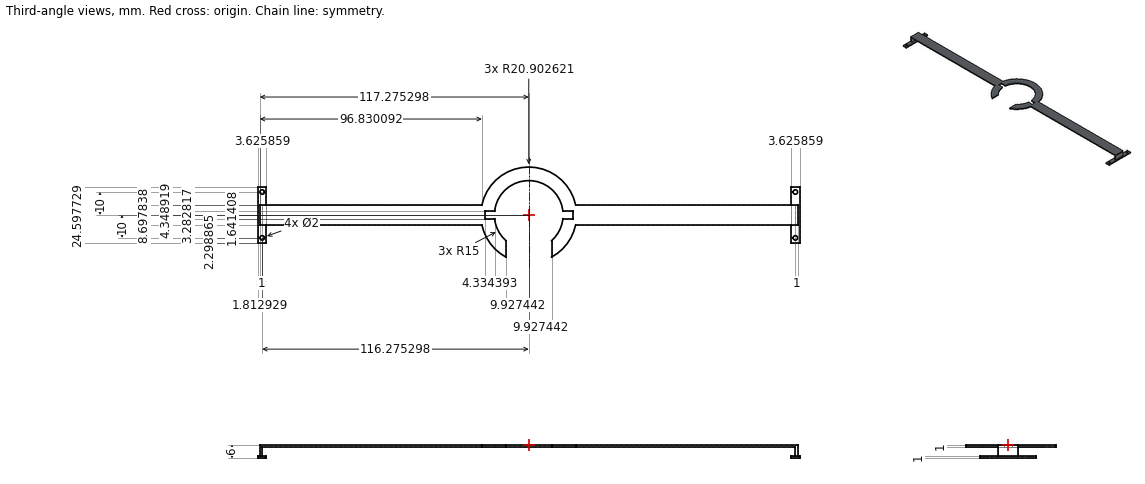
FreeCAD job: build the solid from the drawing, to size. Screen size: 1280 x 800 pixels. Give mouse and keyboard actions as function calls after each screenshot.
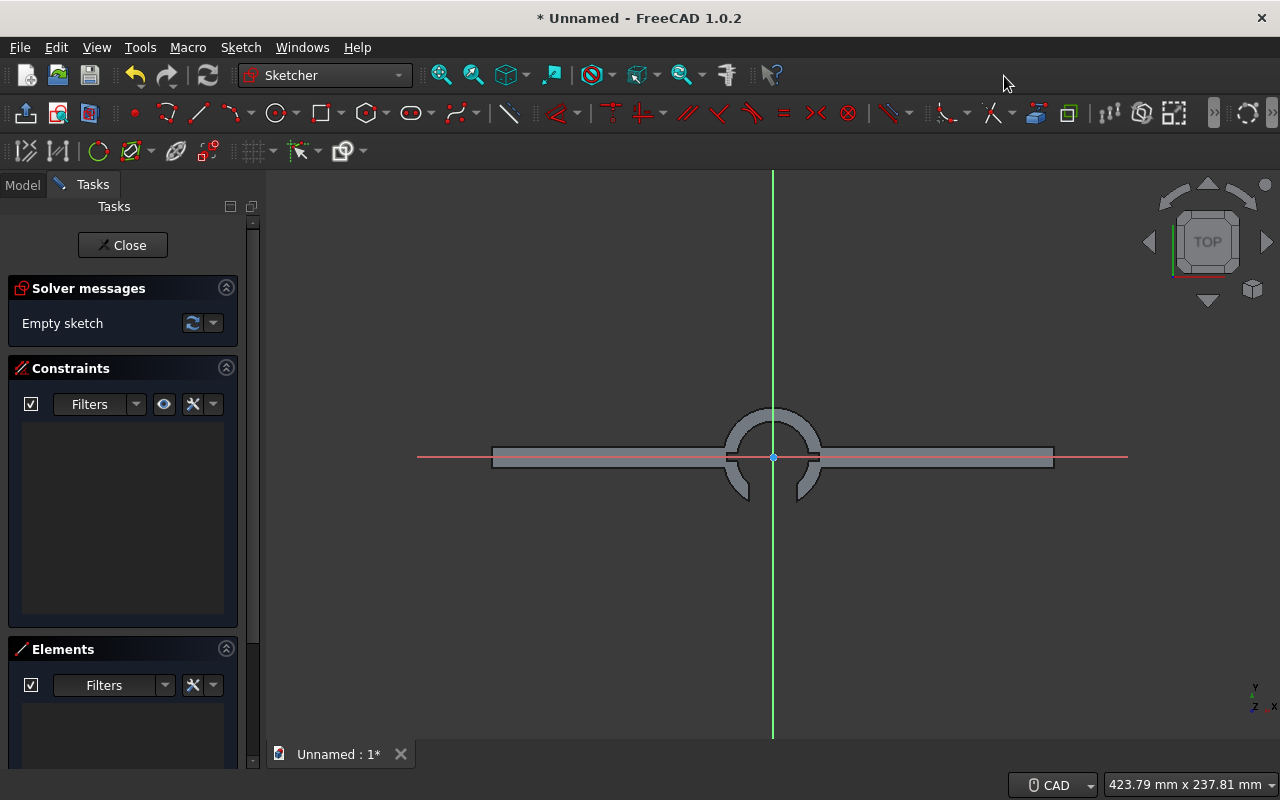
click(322, 114)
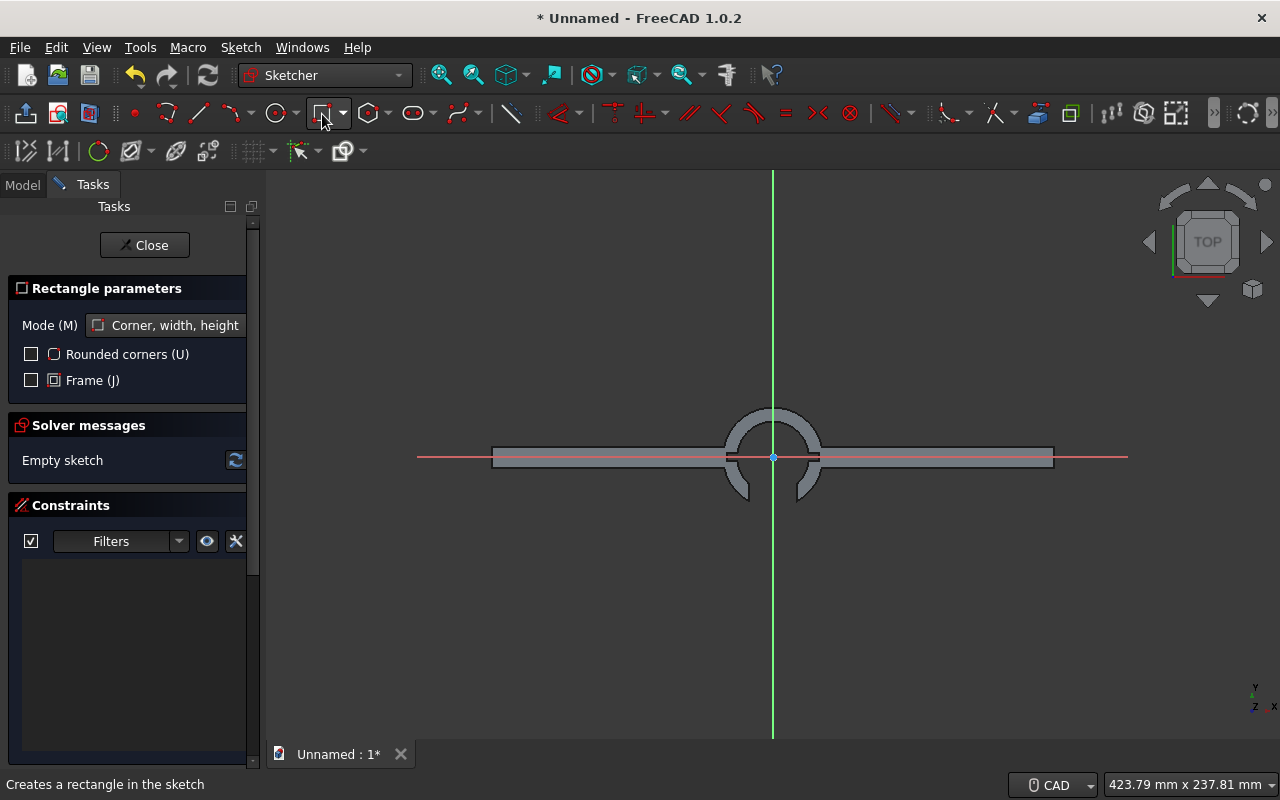
scroll(492, 447, up, 10)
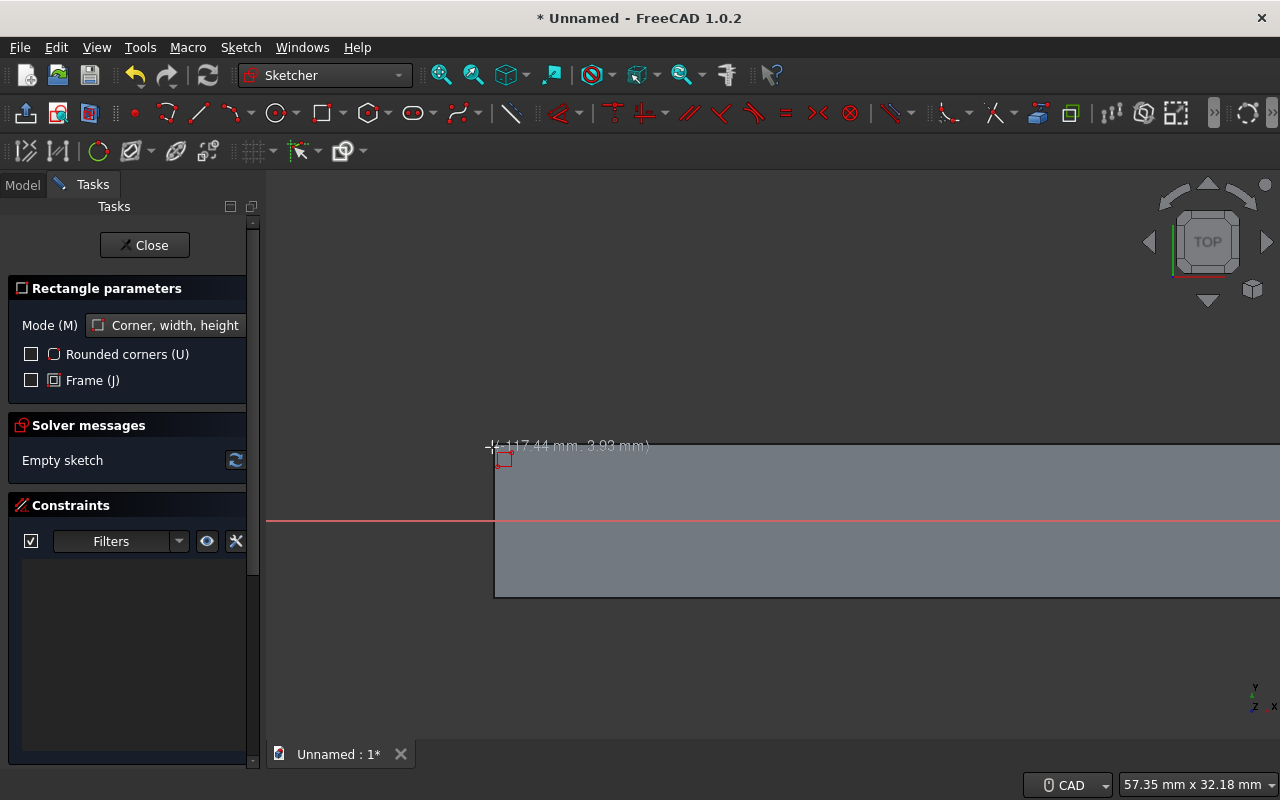
scroll(413, 444, down, 10)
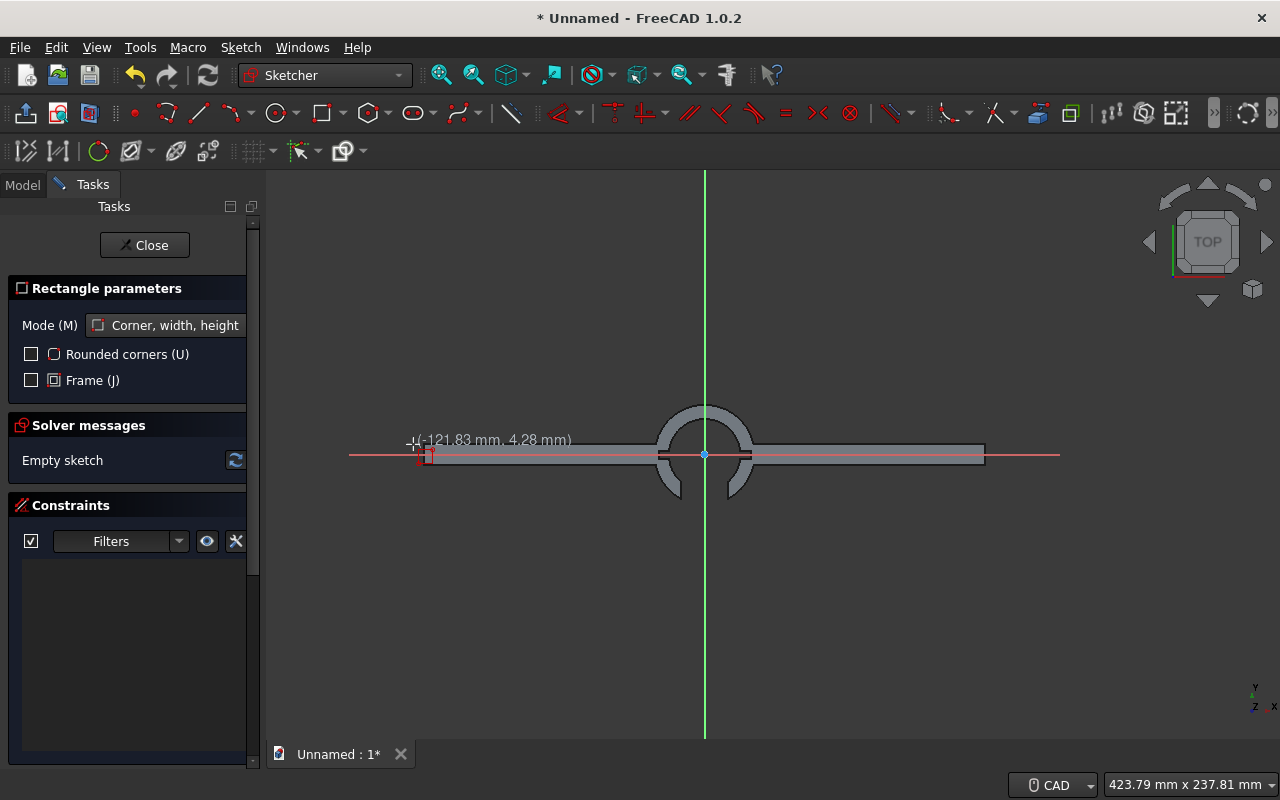
scroll(424, 444, up, 3)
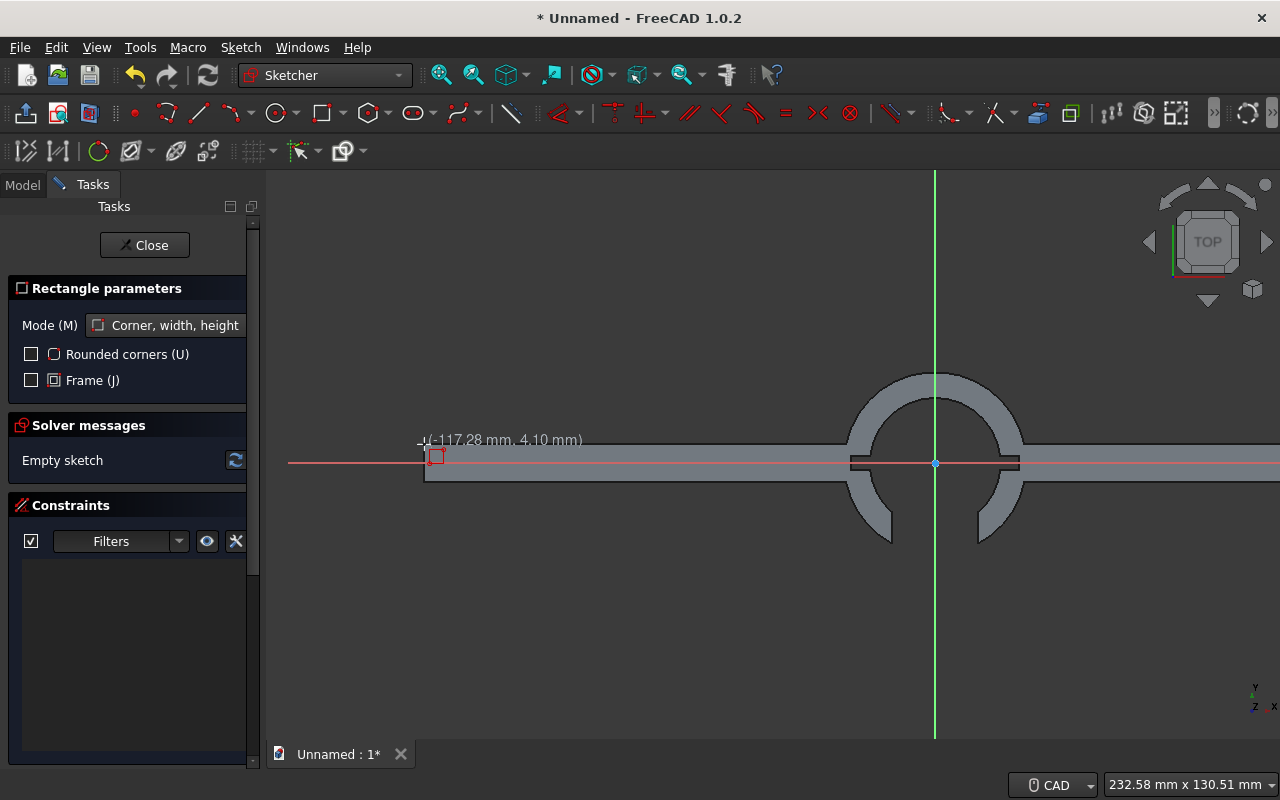
click(424, 444)
move(428, 482)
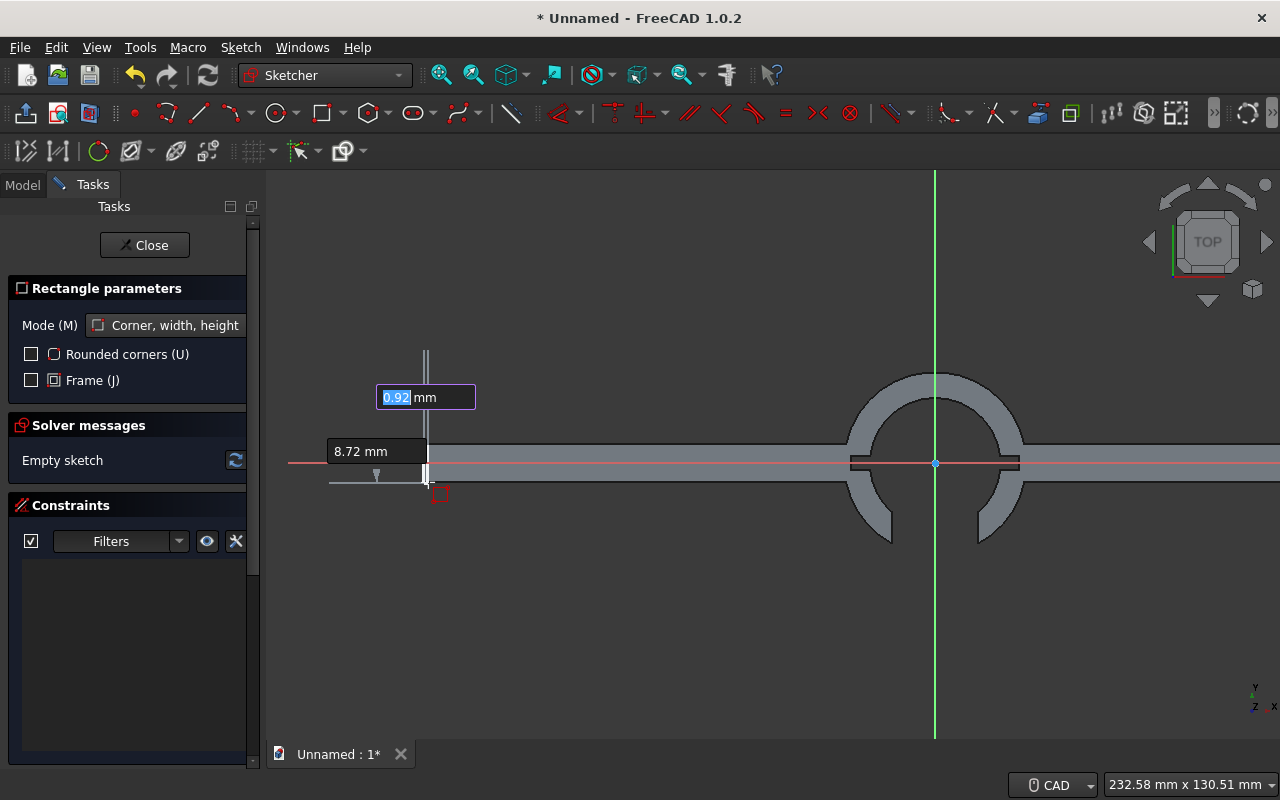
text(1)
key(Tab)
text(8.697838)
key(Return)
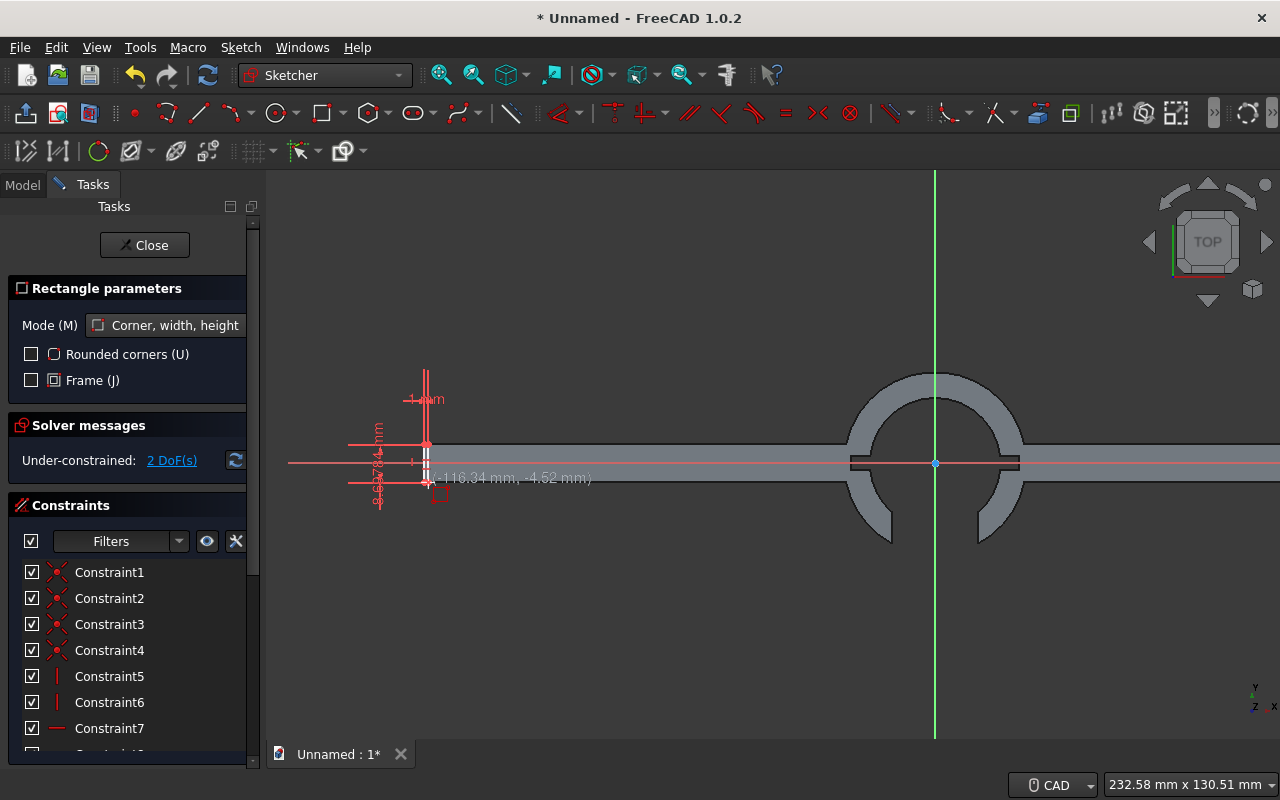
scroll(424, 444, down, 3)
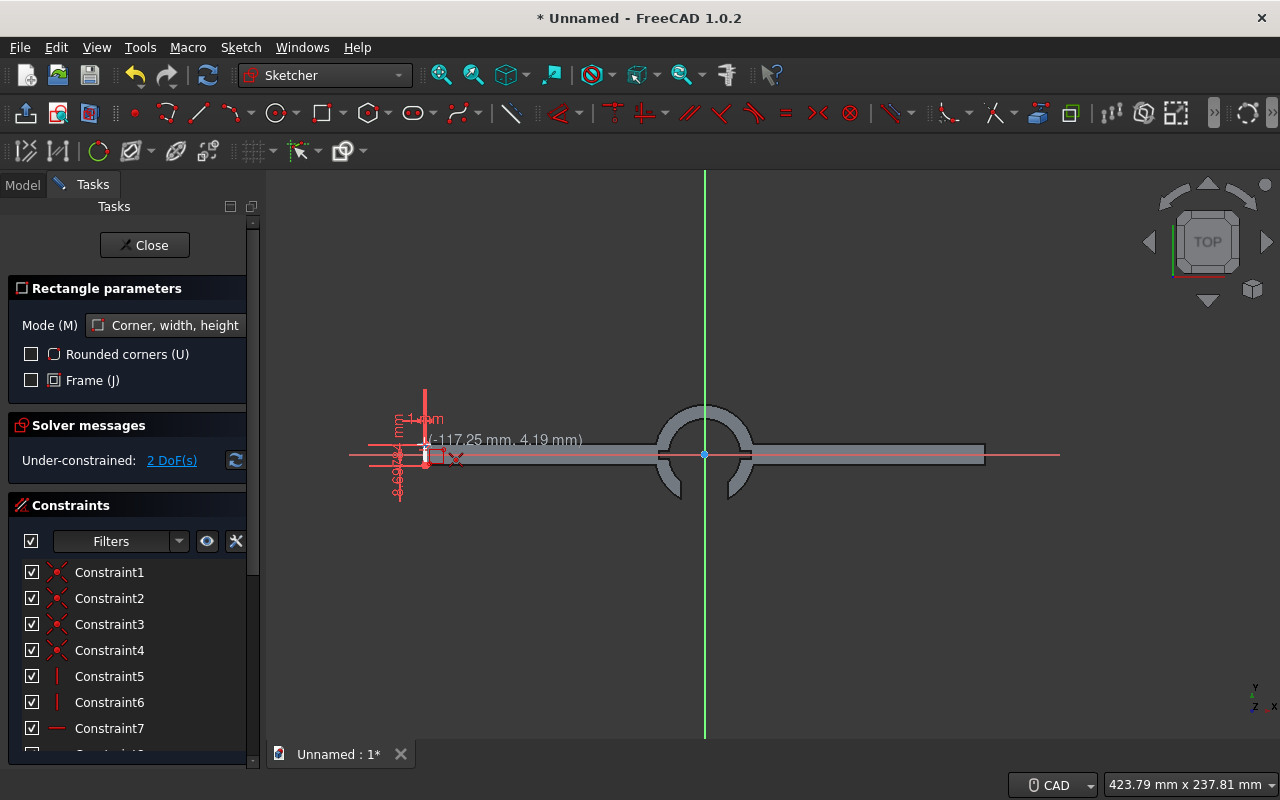
scroll(983, 444, up, 10)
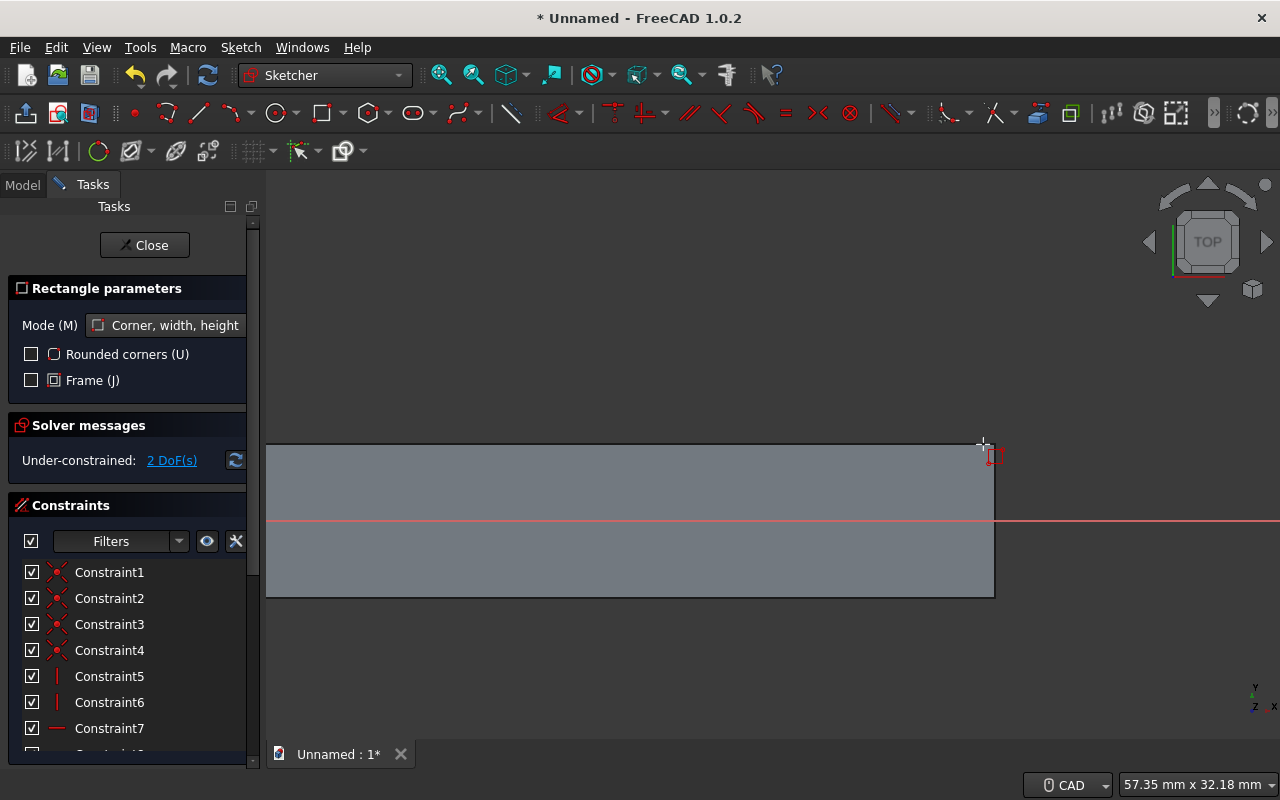
scroll(984, 444, down, 10)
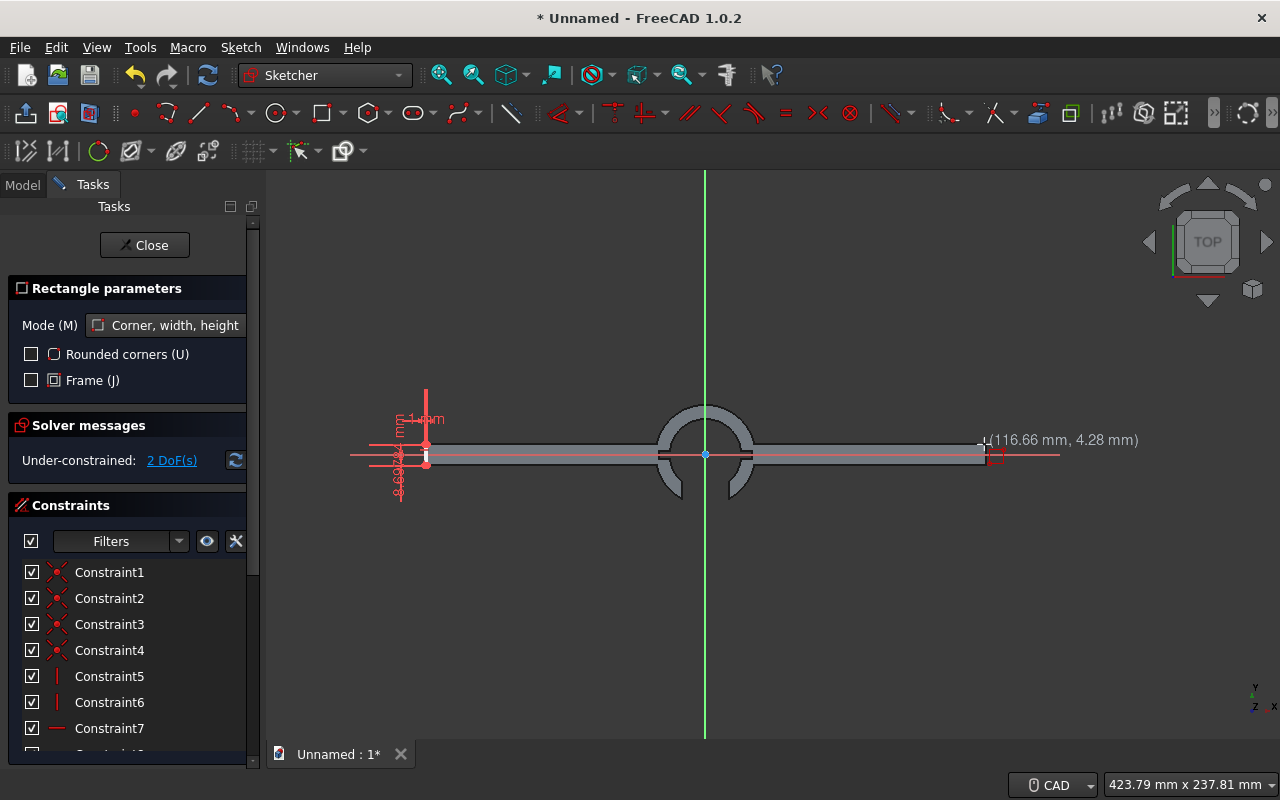
scroll(984, 444, up, 3)